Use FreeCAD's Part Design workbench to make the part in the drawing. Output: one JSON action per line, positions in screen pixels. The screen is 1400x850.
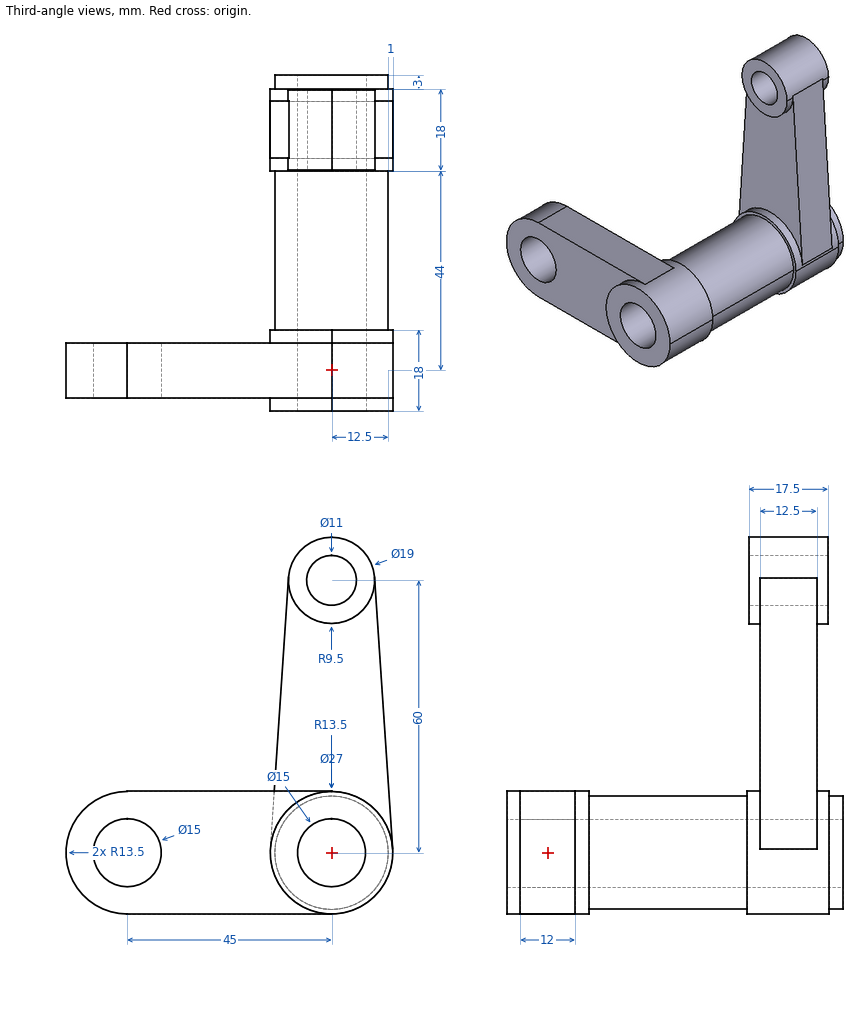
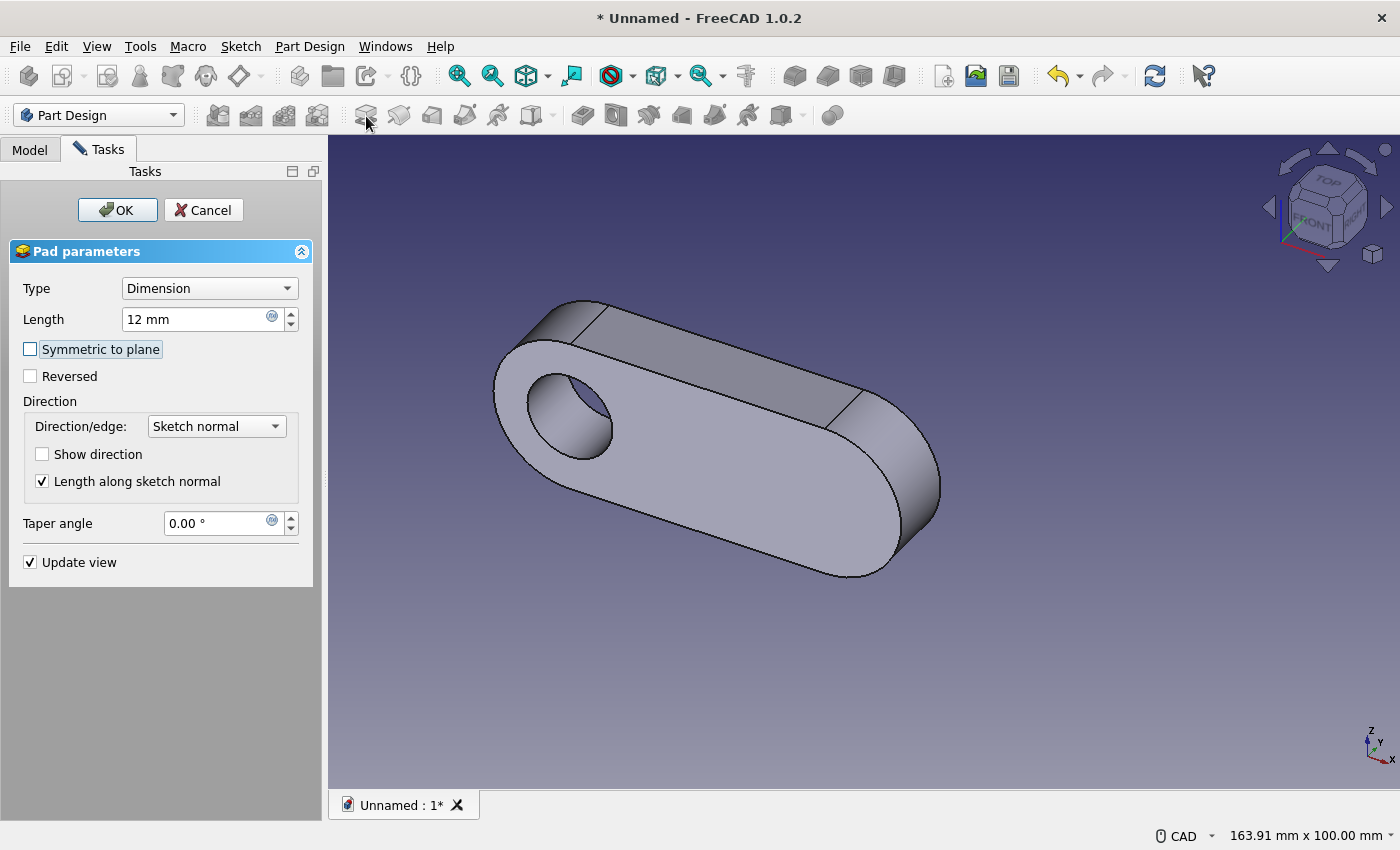
{"action": "left_click", "coordinate": [31, 349]}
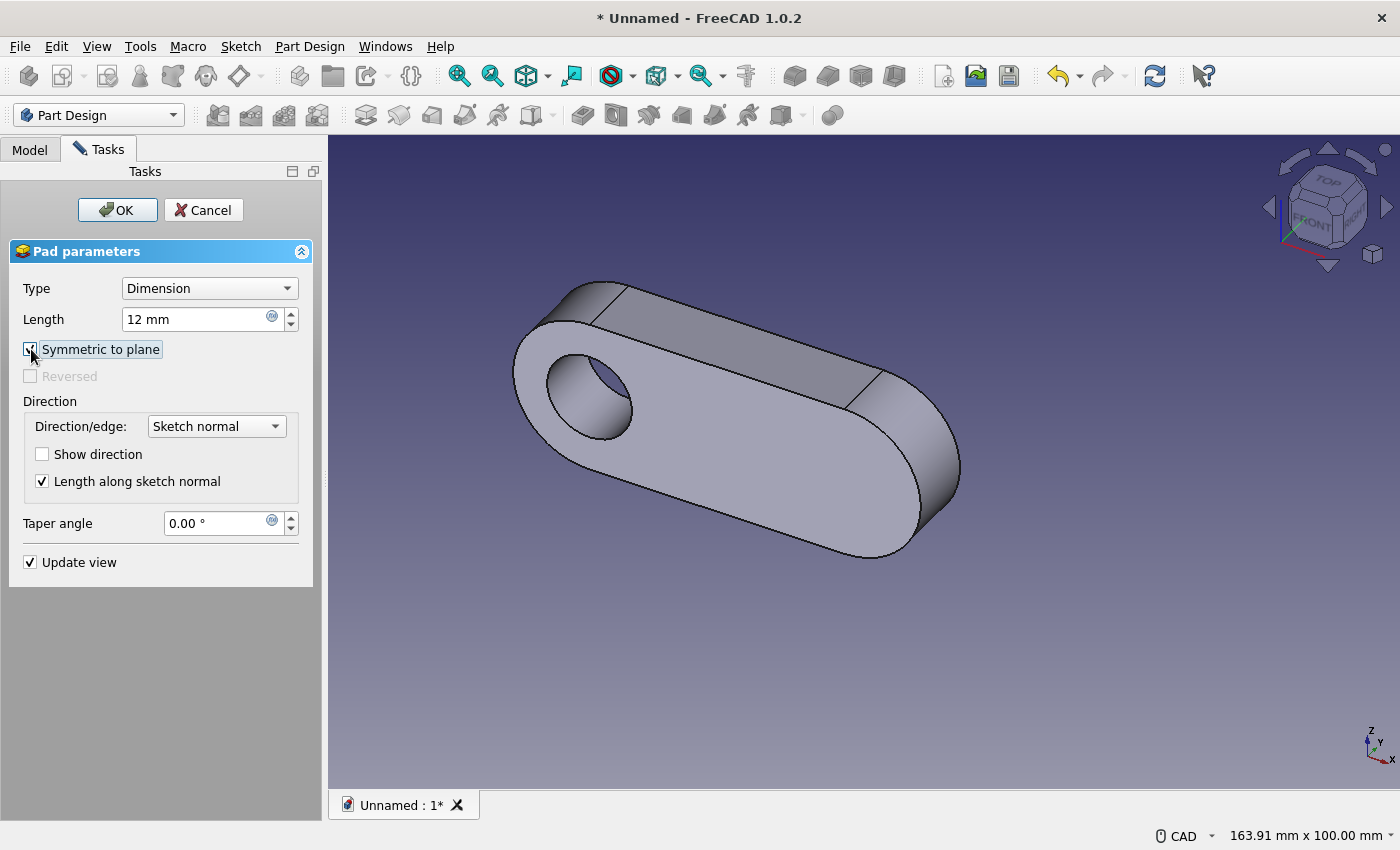
{"action": "left_click", "coordinate": [118, 210]}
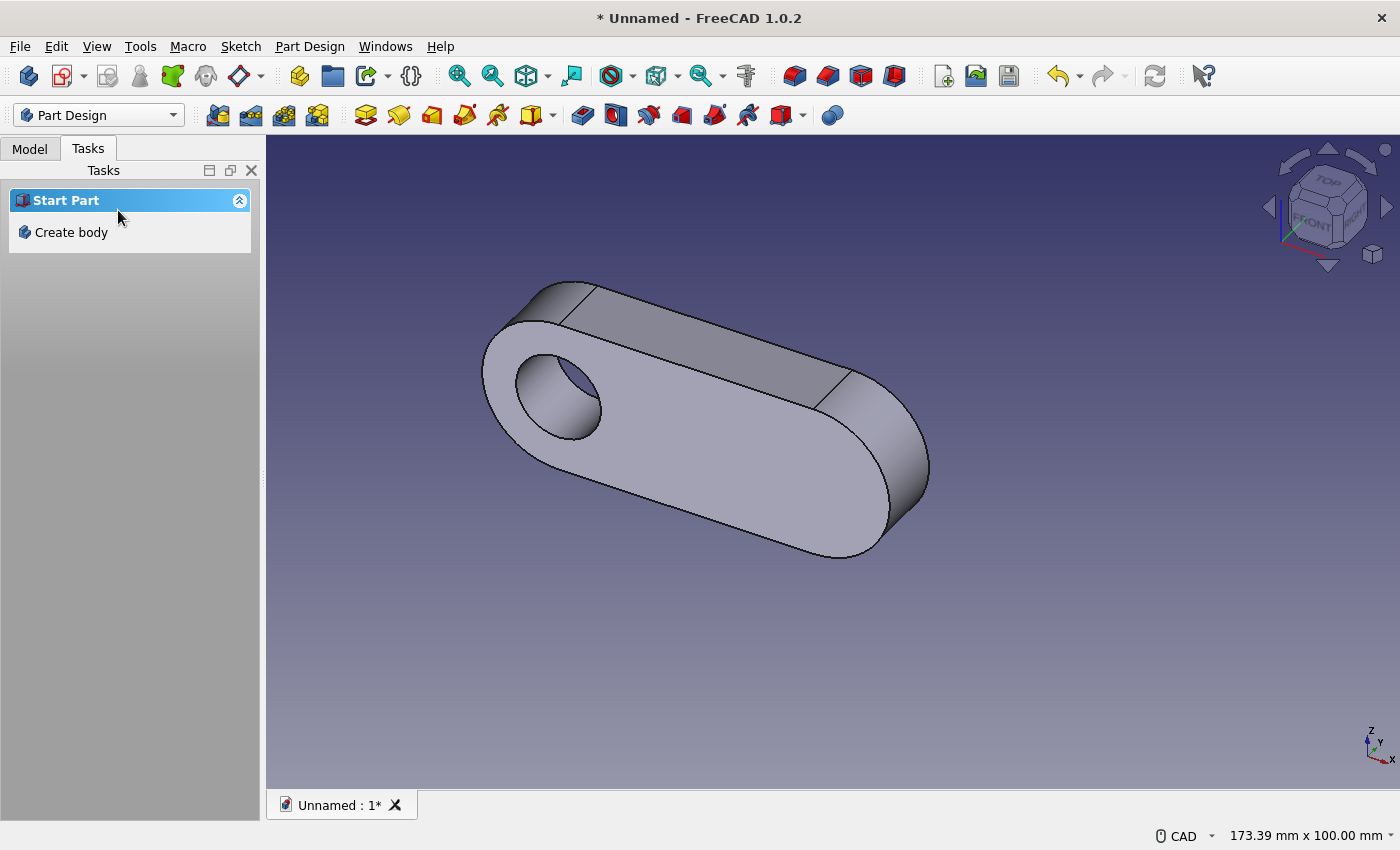
{"action": "left_click", "coordinate": [62, 76]}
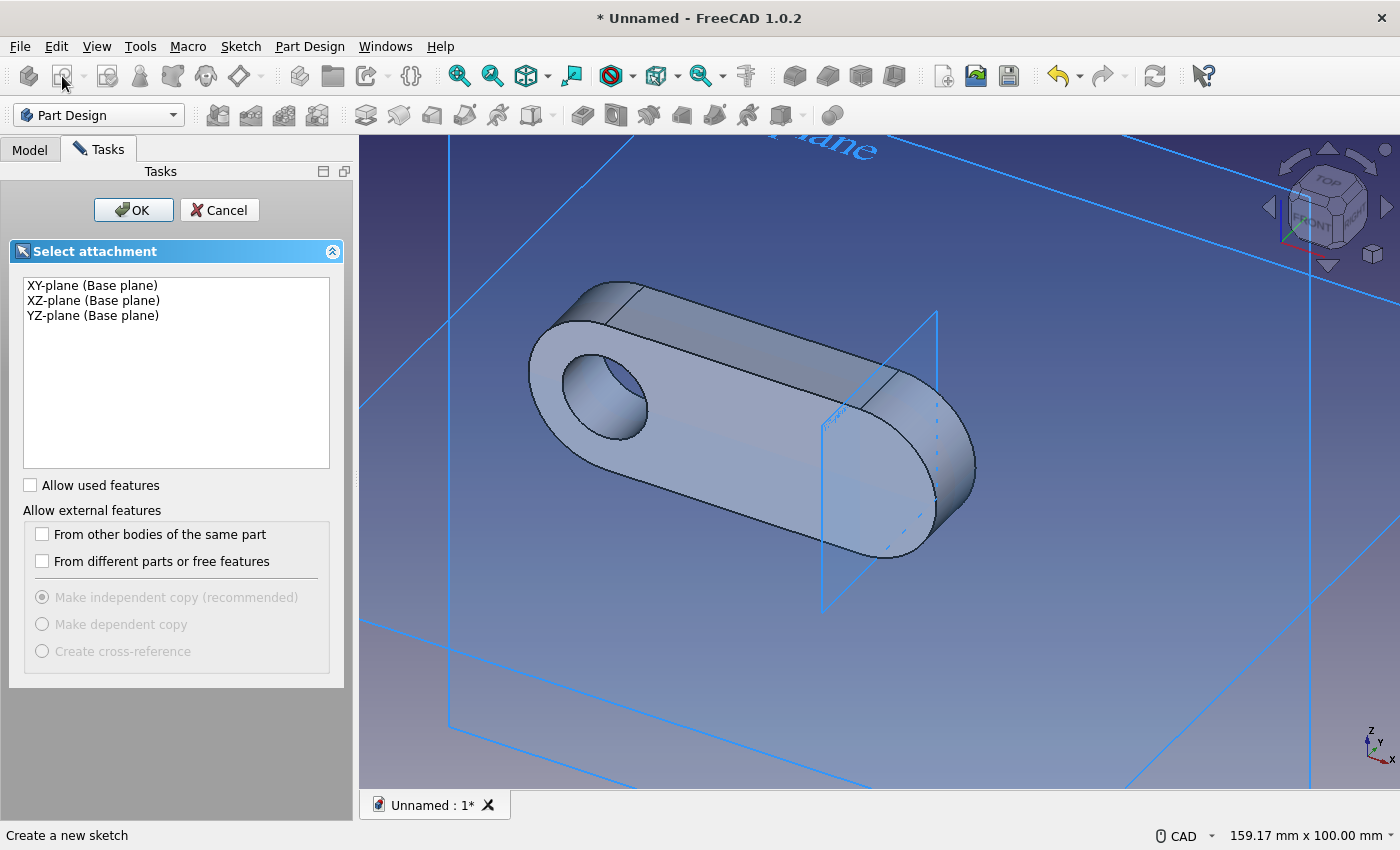
{"action": "left_click", "coordinate": [84, 300]}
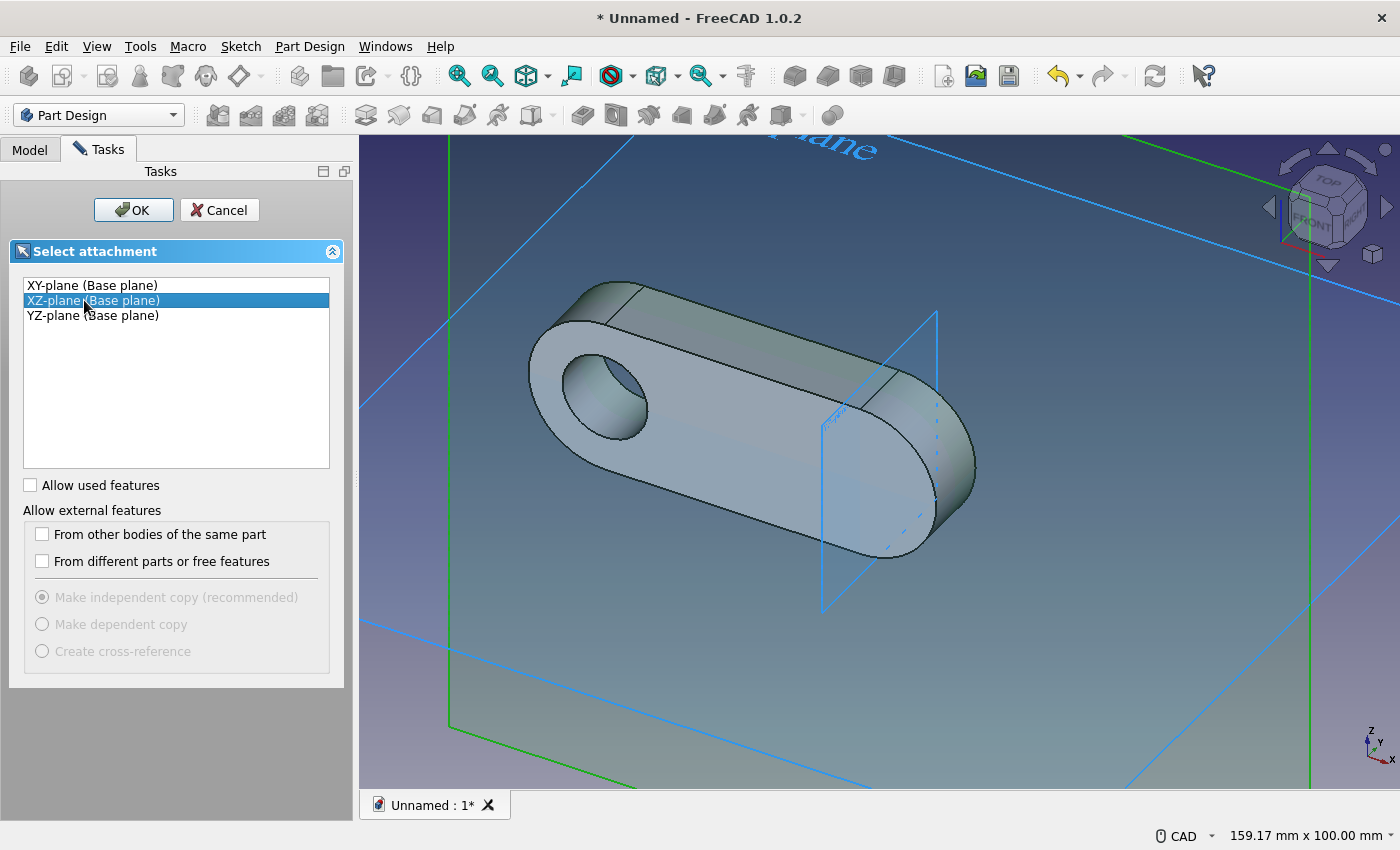
{"action": "left_click", "coordinate": [134, 210]}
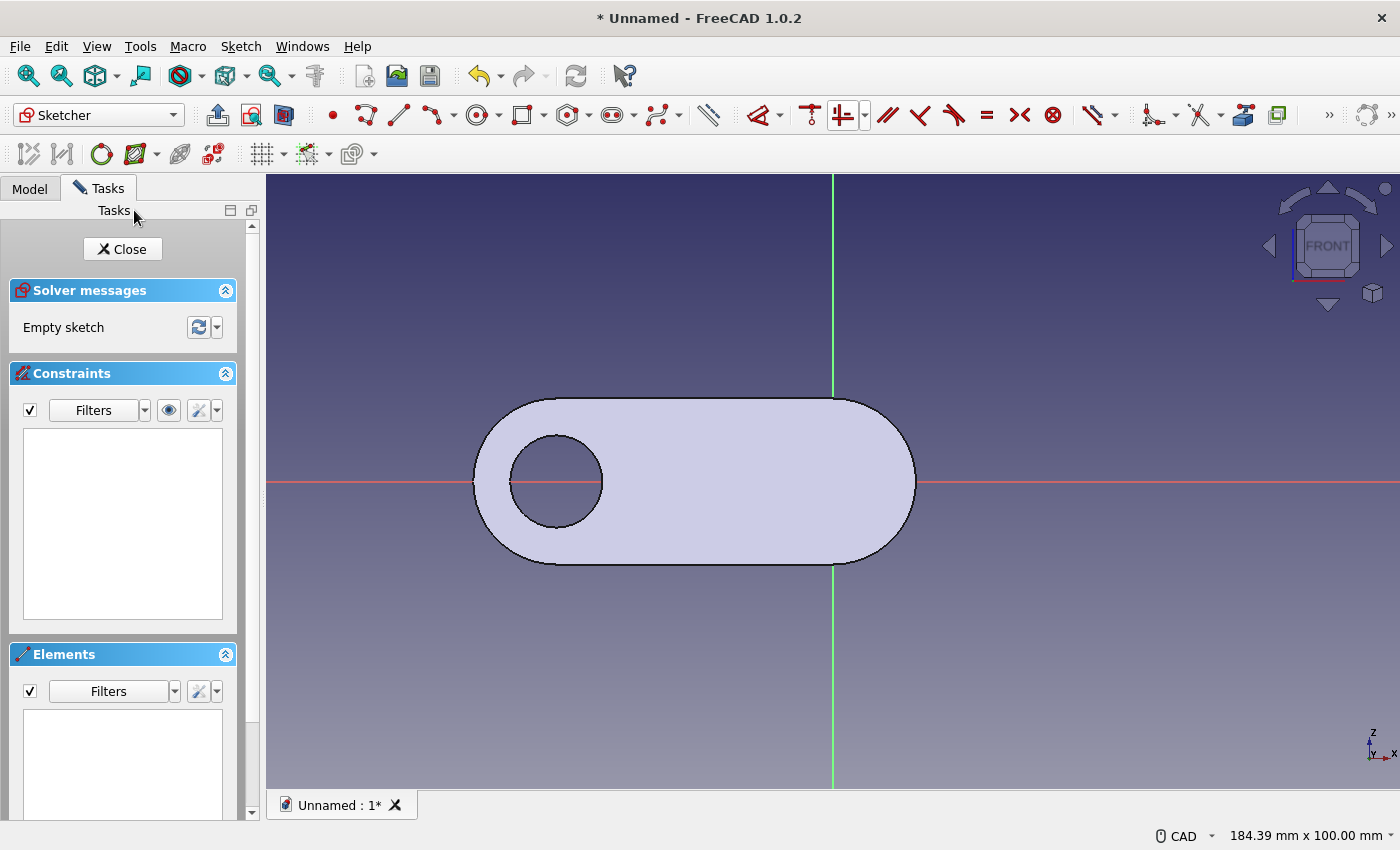
{"action": "left_click", "coordinate": [284, 116]}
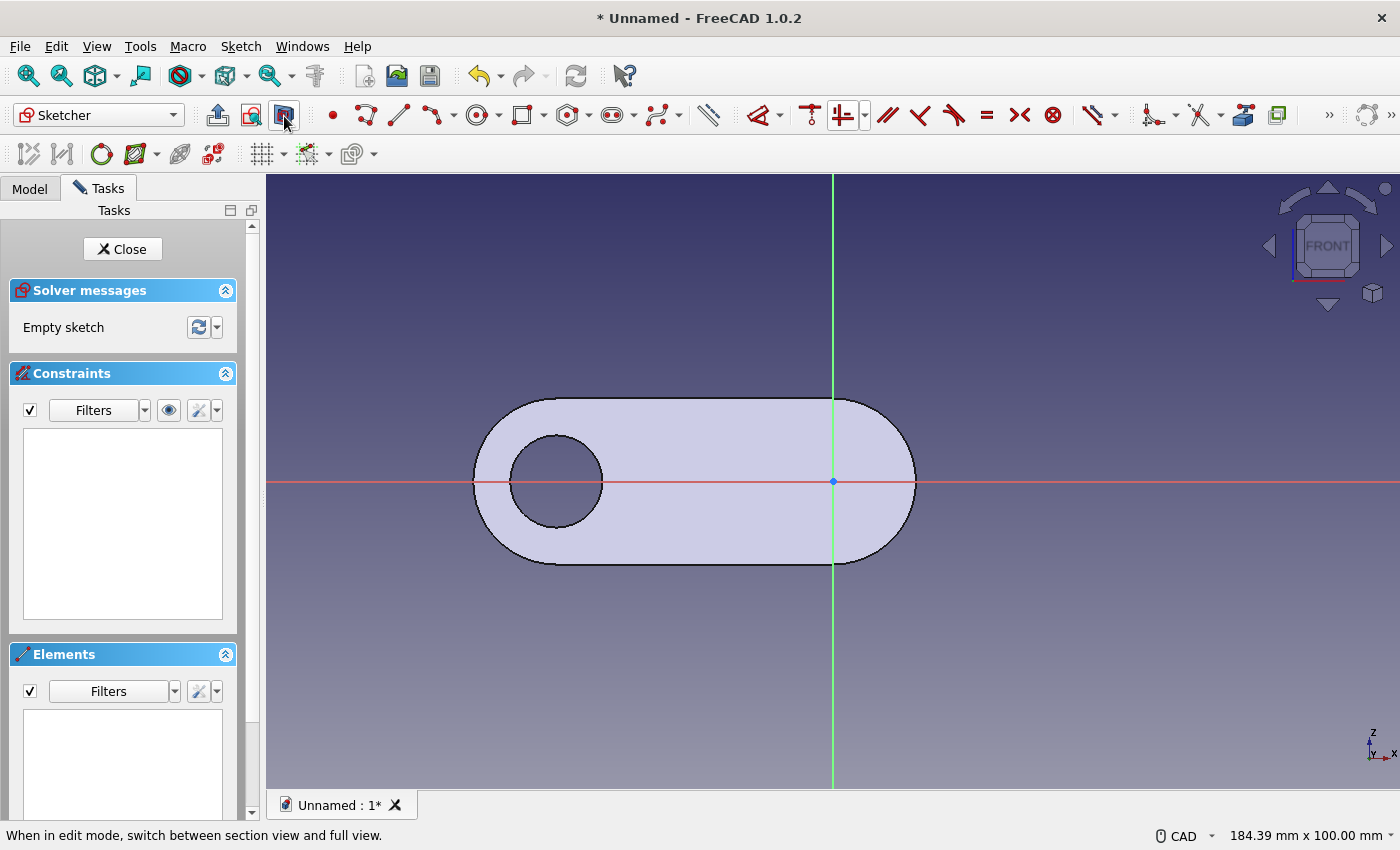
{"action": "scroll", "coordinate": [889, 482], "scroll_direction": "up", "scroll_amount": 4}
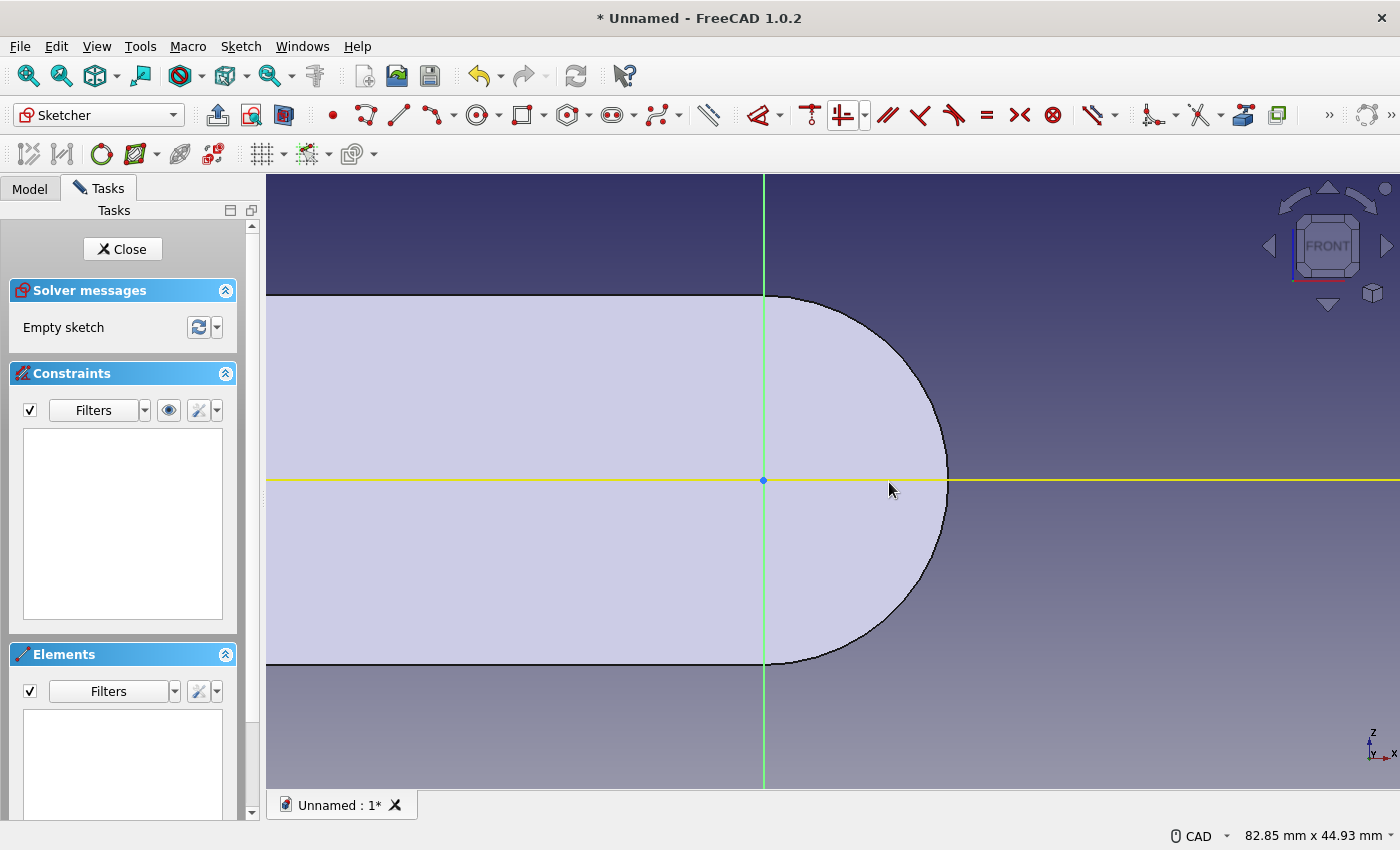
{"action": "left_click", "coordinate": [476, 116]}